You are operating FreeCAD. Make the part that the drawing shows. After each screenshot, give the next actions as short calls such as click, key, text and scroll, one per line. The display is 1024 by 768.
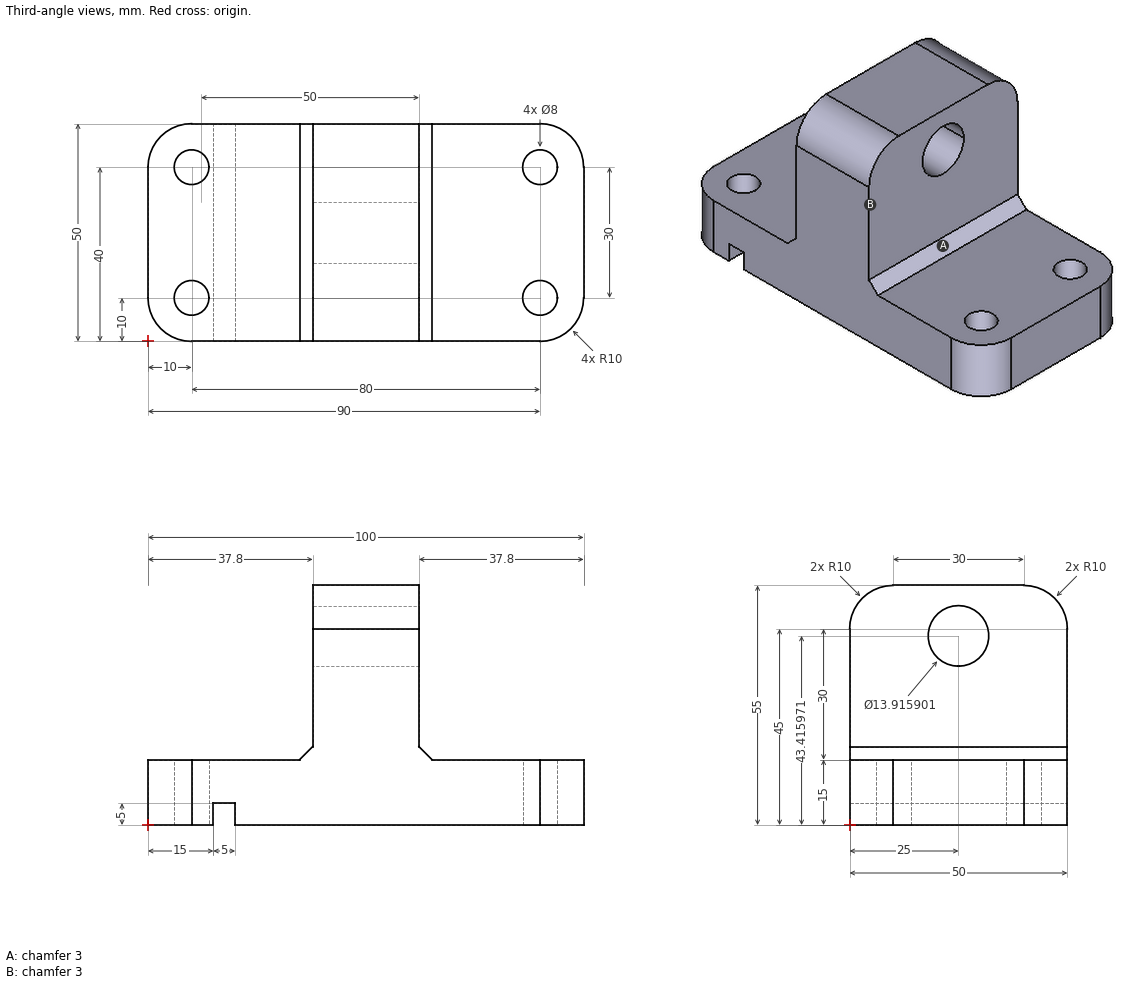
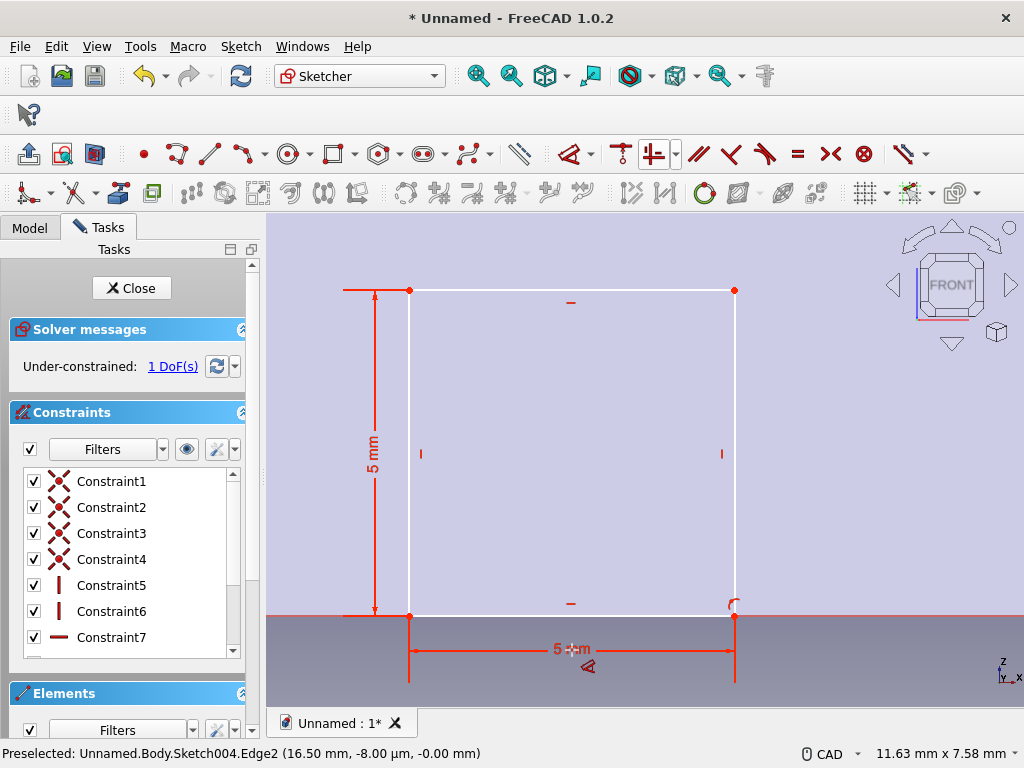
click(409, 290)
click(352, 650)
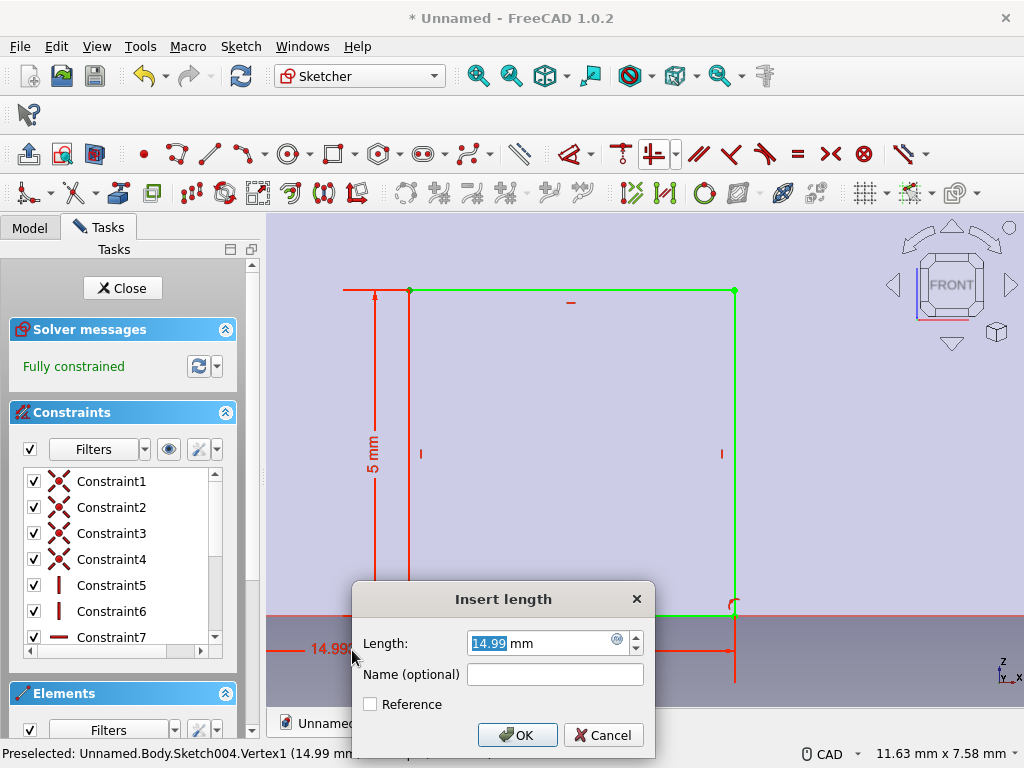
text(15)
key(Return)
key(Escape)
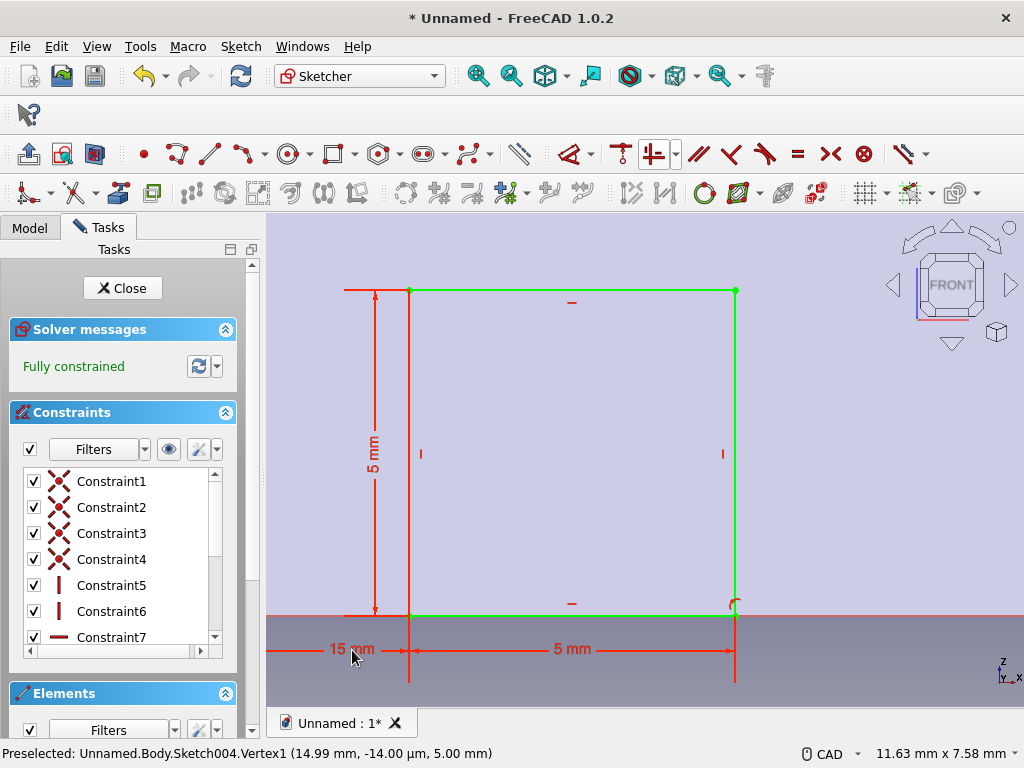
click(123, 288)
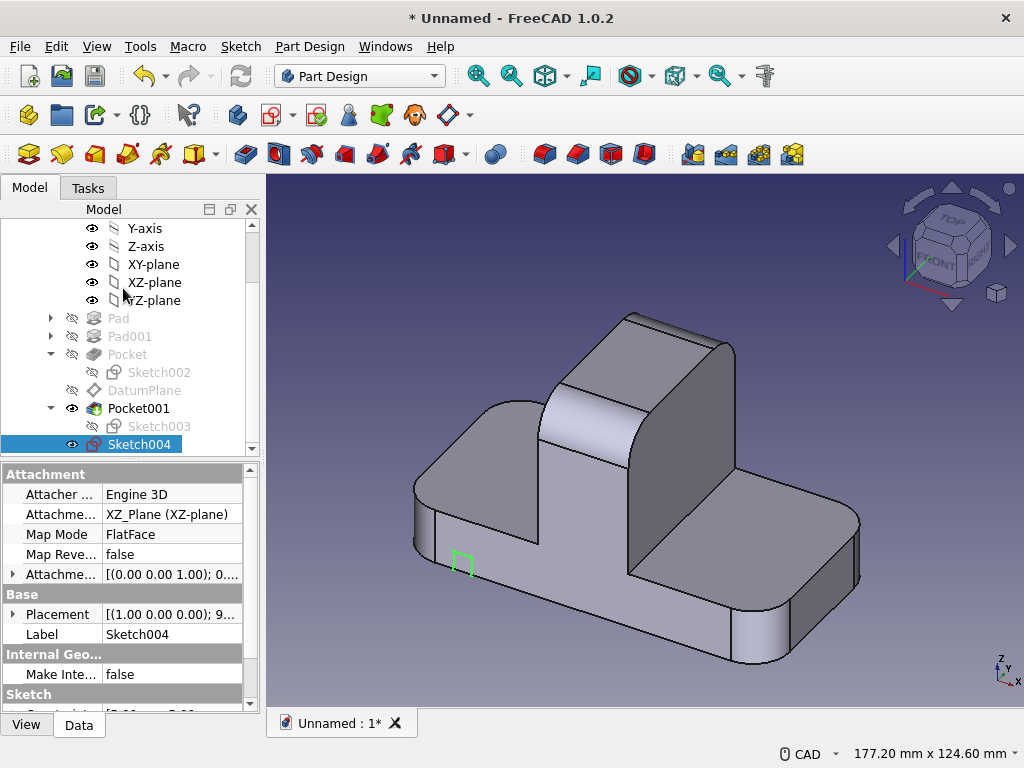
click(246, 154)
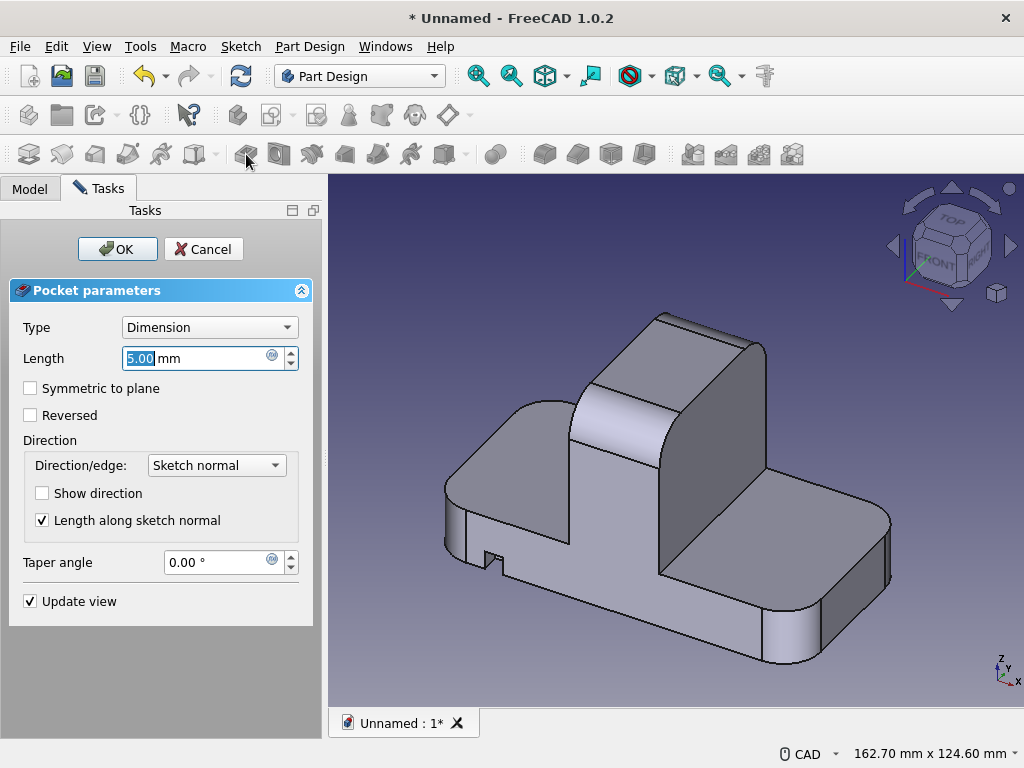
text(50)
key(Tab)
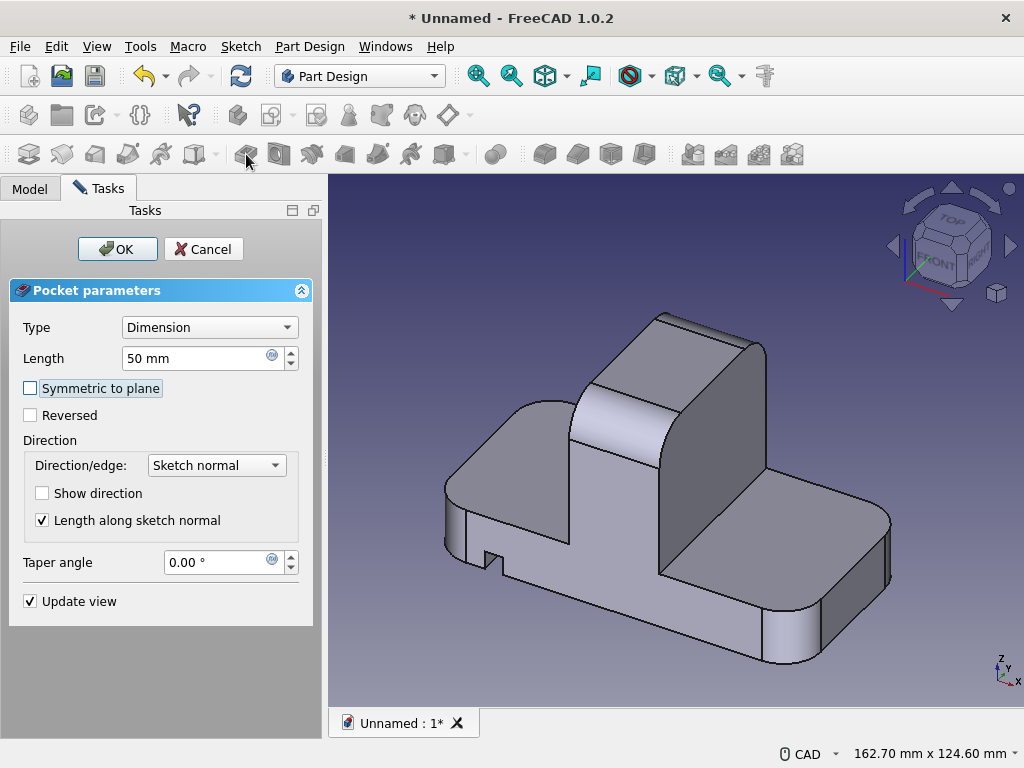
click(118, 249)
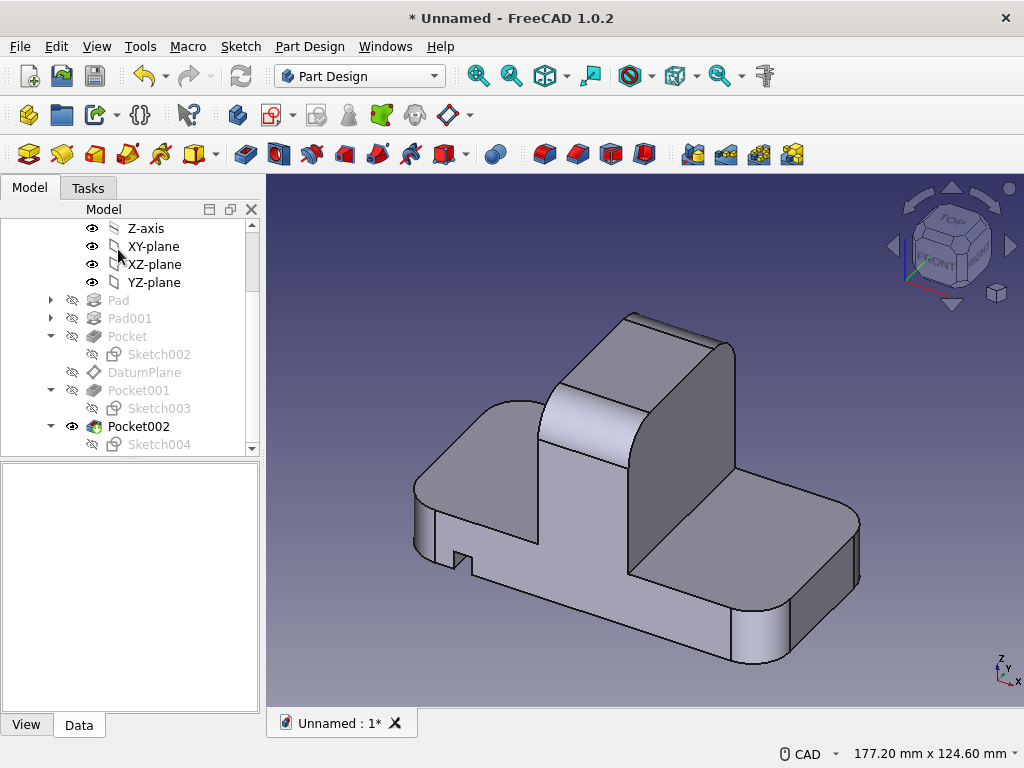
click(682, 450)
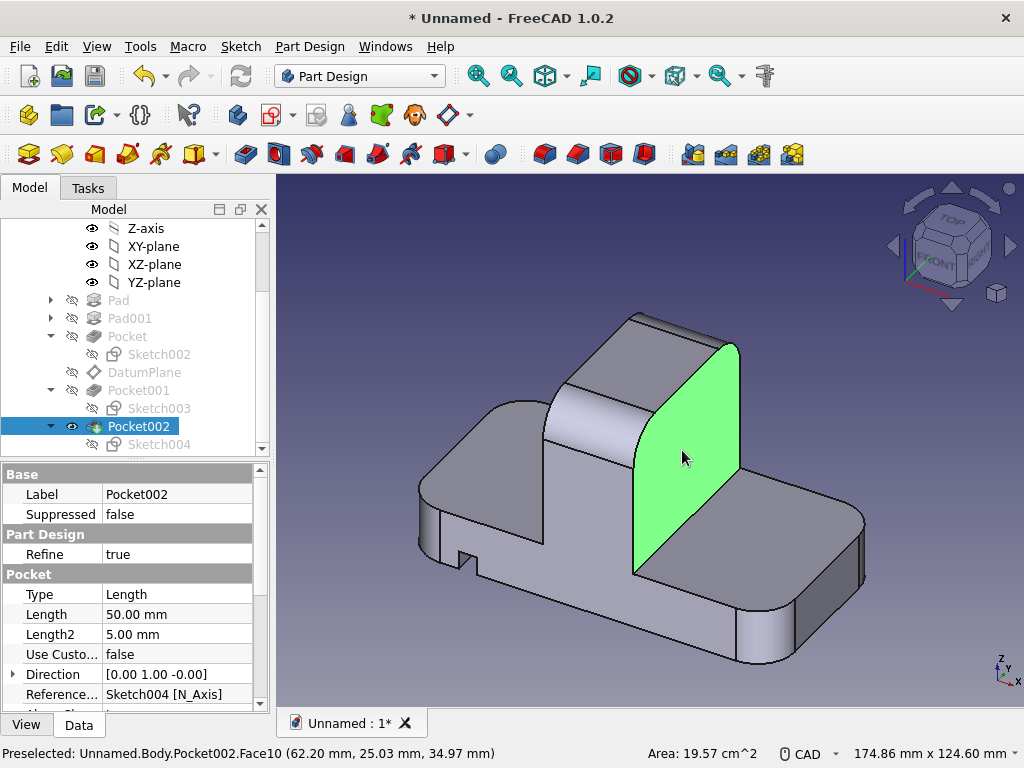
click(270, 116)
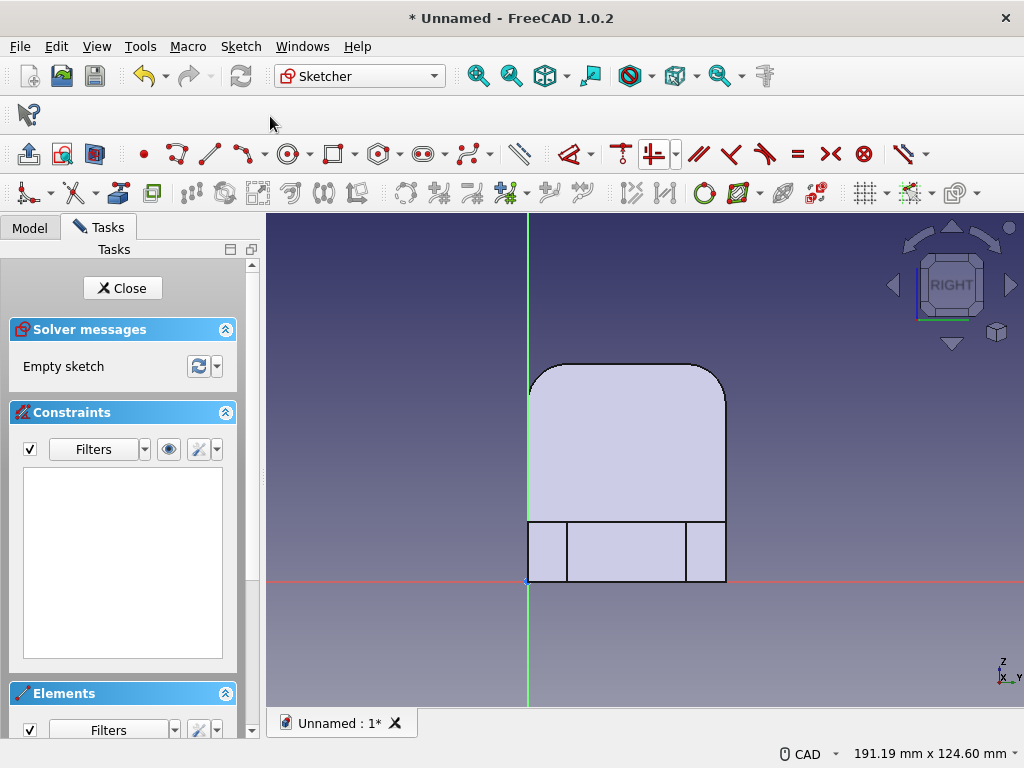
scroll(637, 400, up, 9)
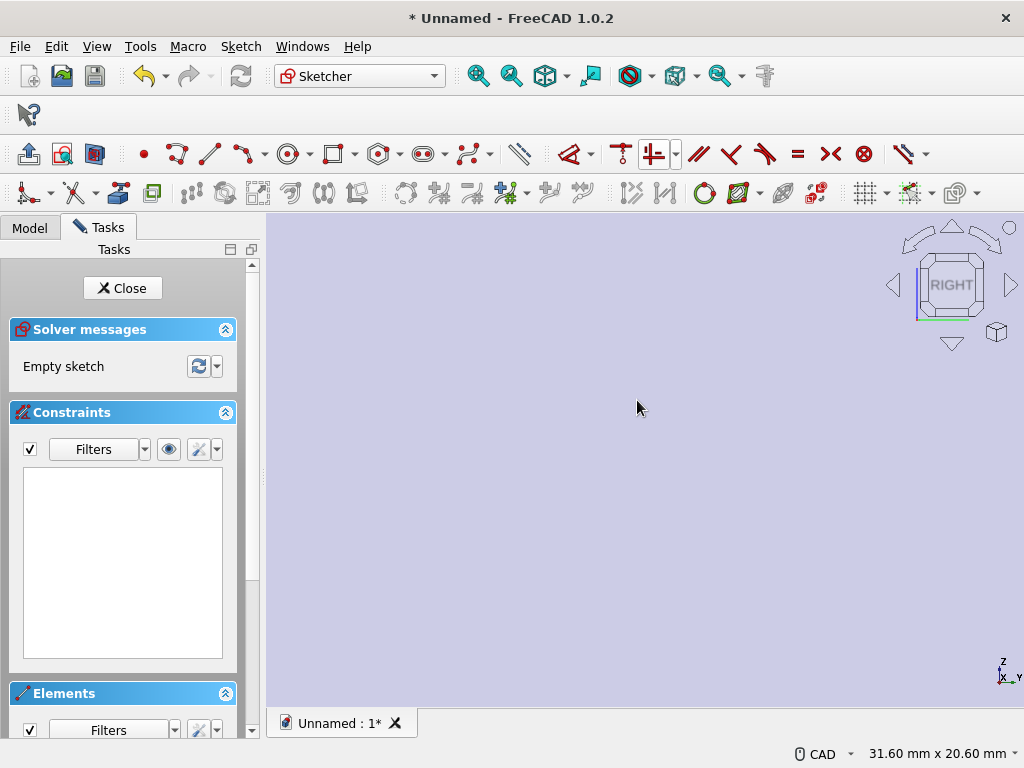
click(288, 154)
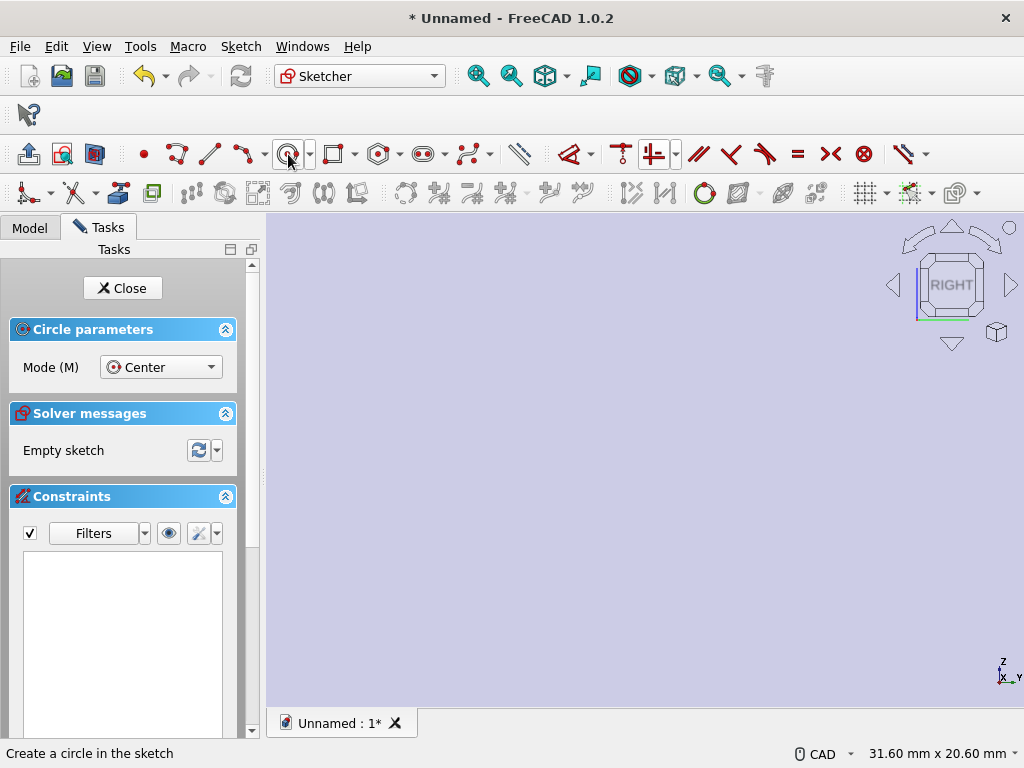
click(572, 458)
click(690, 340)
key(Escape)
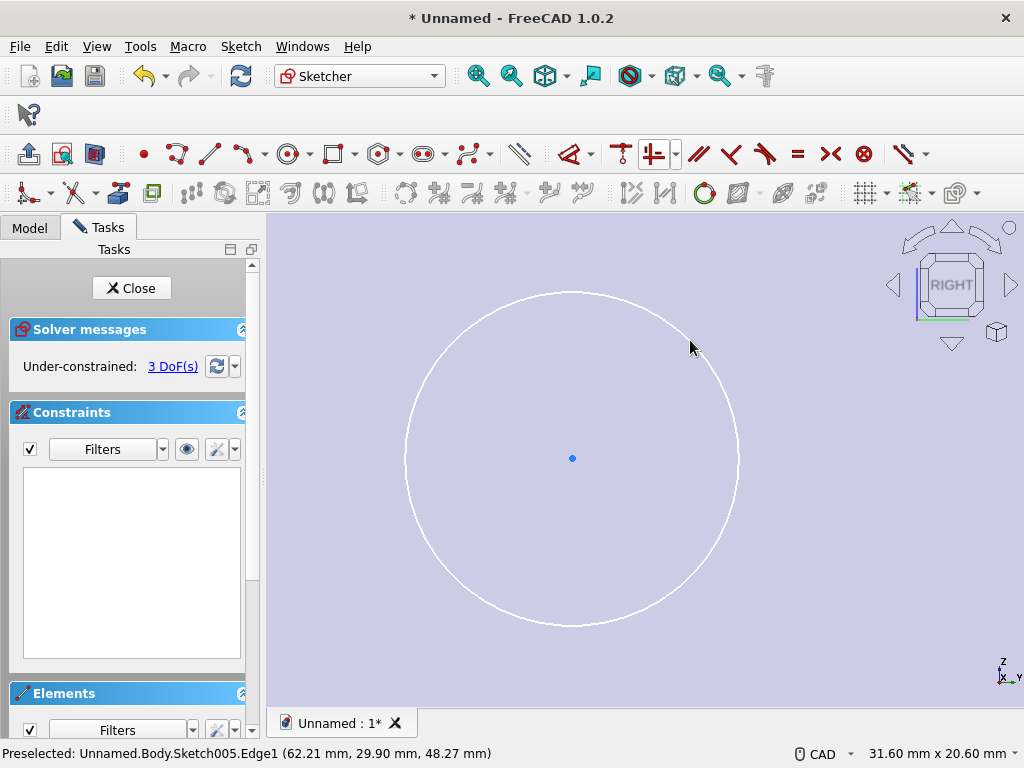
click(568, 154)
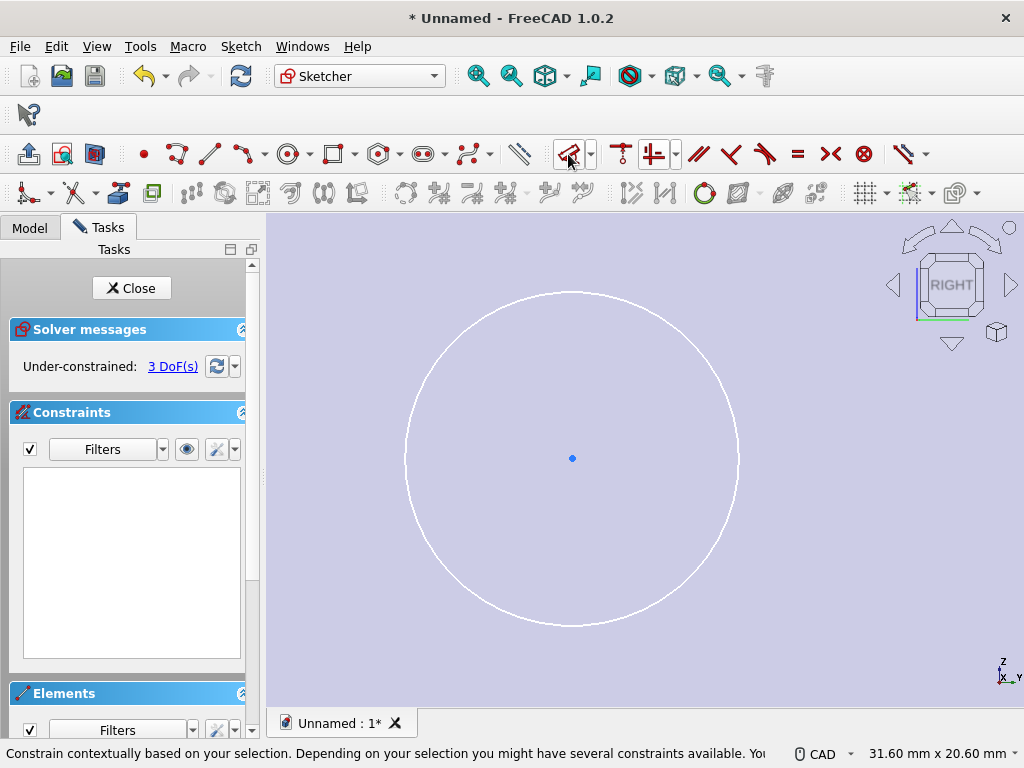
click(690, 341)
click(713, 318)